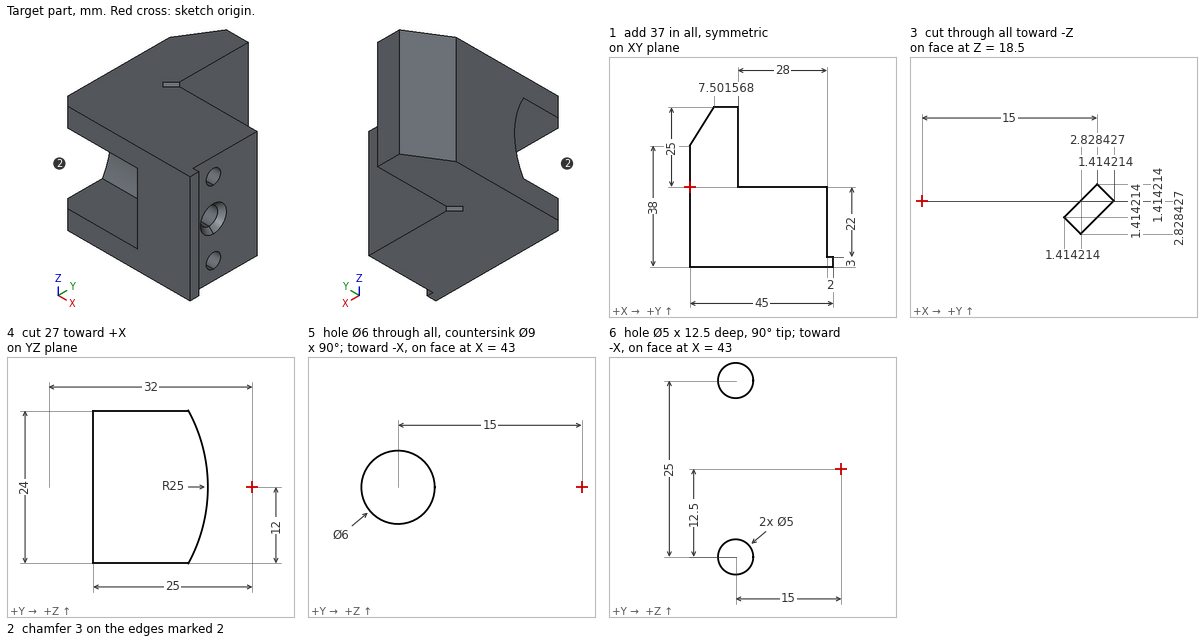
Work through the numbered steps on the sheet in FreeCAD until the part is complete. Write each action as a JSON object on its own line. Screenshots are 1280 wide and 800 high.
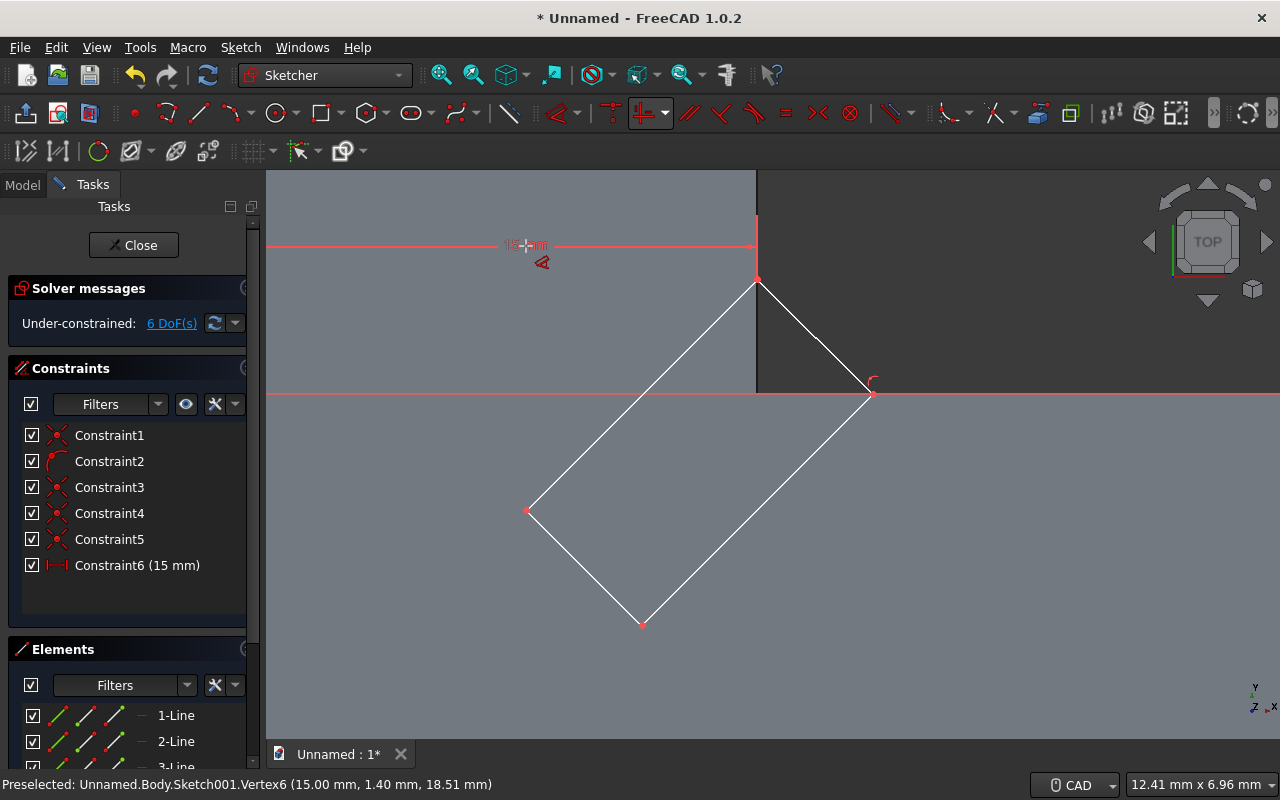
{"action": "left_click", "coordinate": [526, 511]}
{"action": "left_click", "coordinate": [560, 453]}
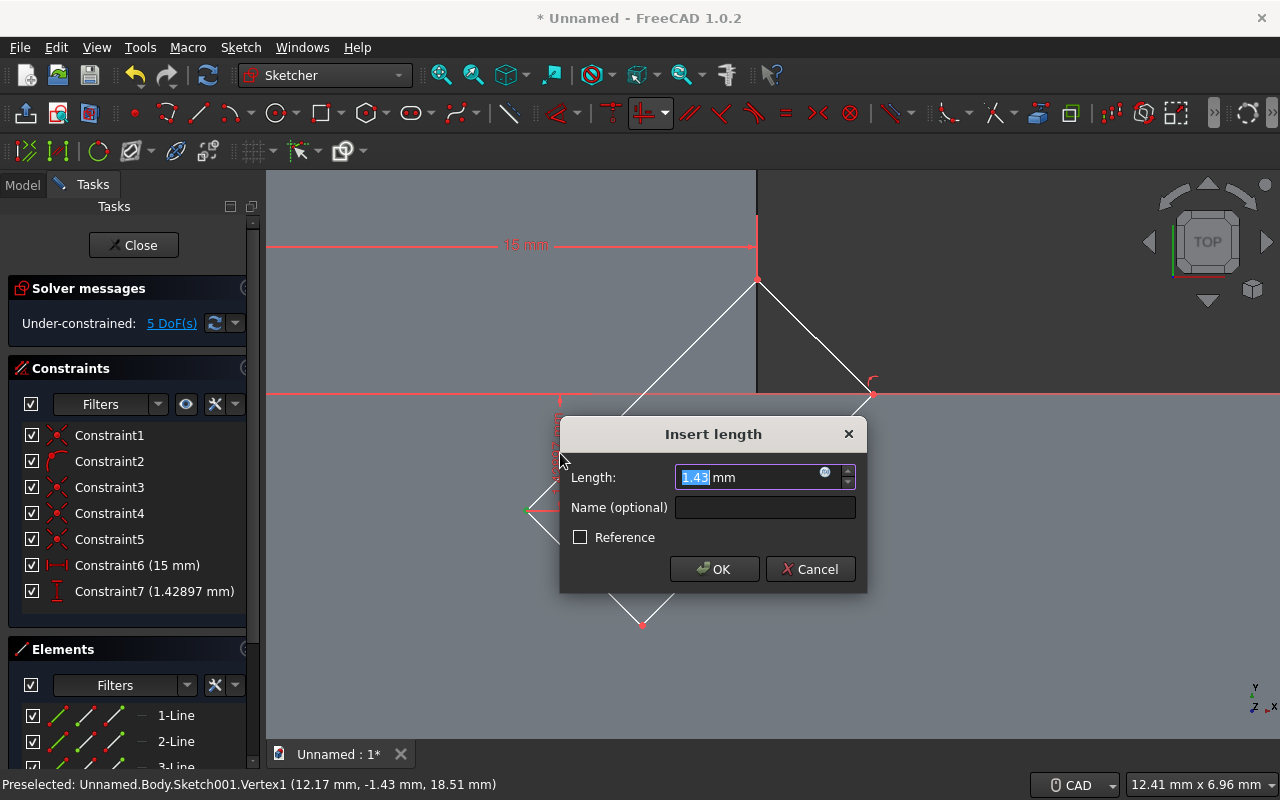
{"action": "type", "text": "1.414214"}
{"action": "key", "text": "Return"}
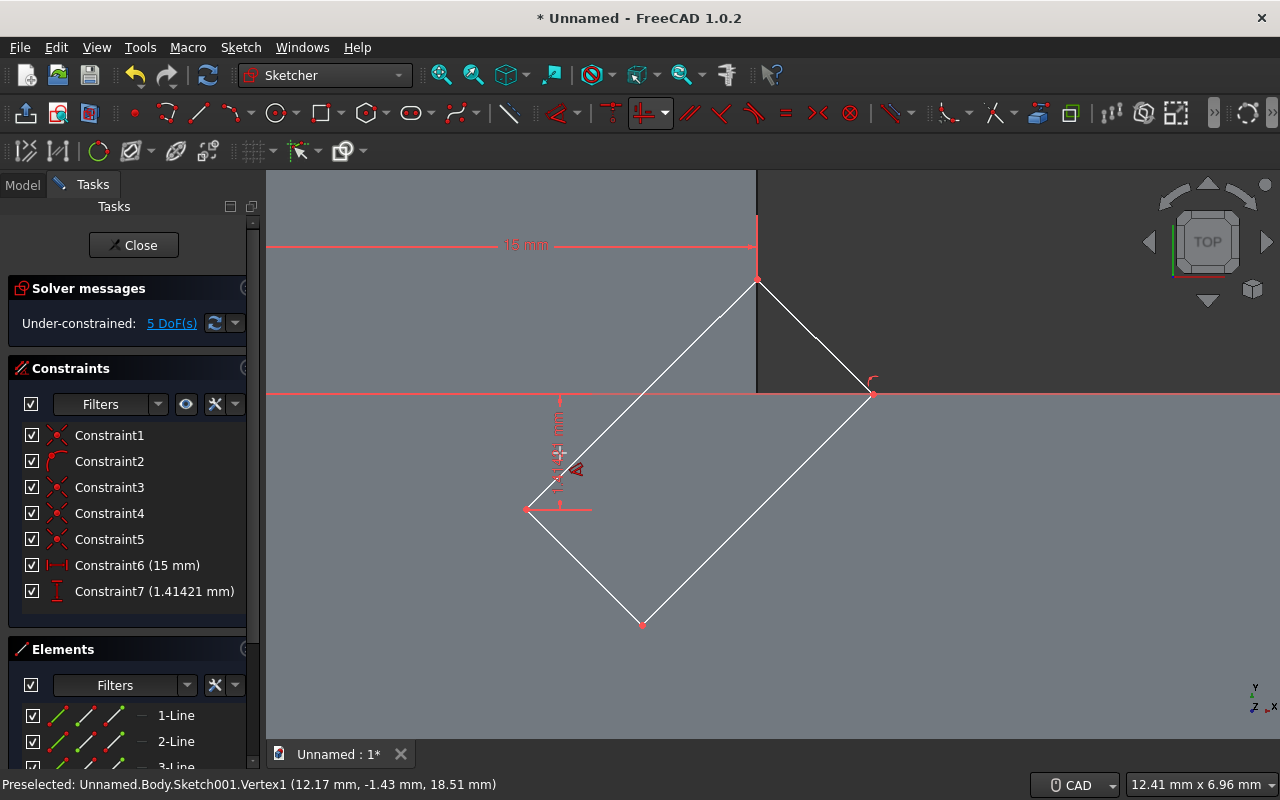
{"action": "left_click", "coordinate": [642, 626]}
{"action": "left_click", "coordinate": [676, 510]}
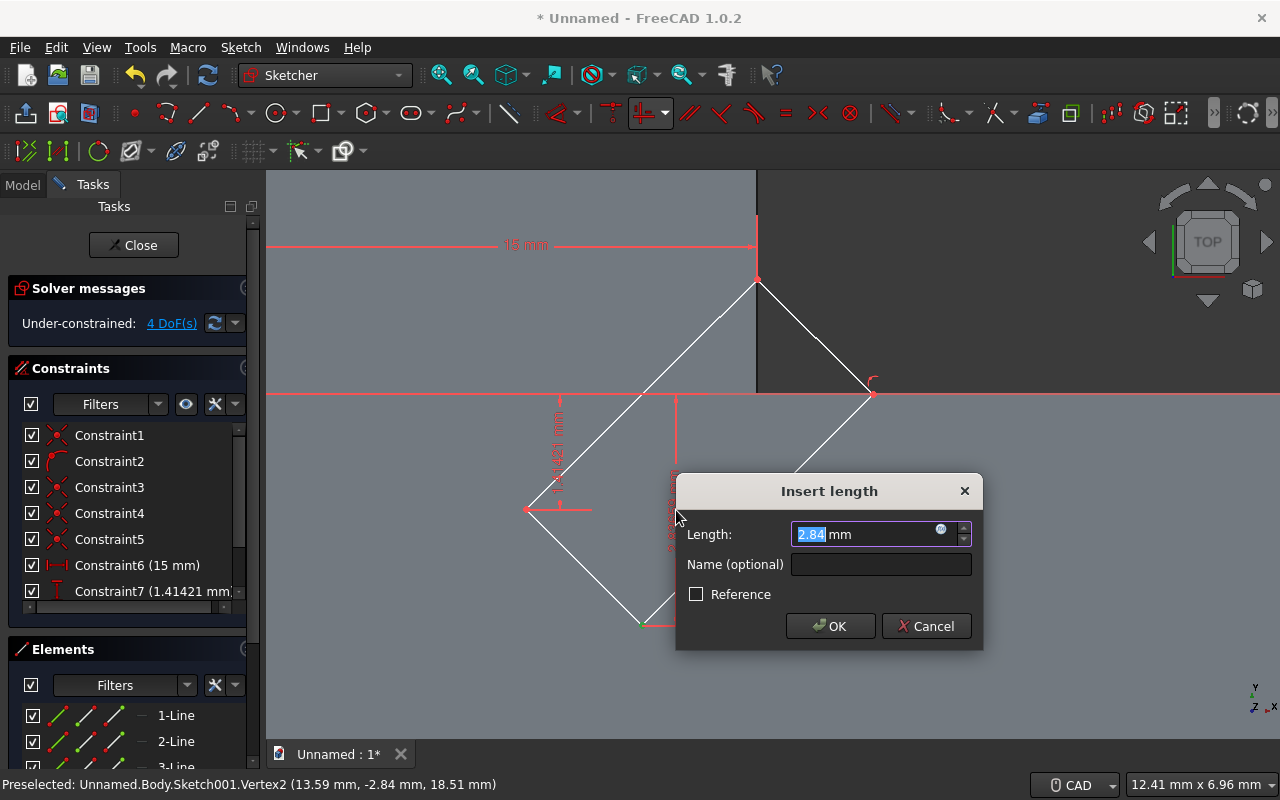
{"action": "type", "text": "2.828427"}
{"action": "key", "text": "Return"}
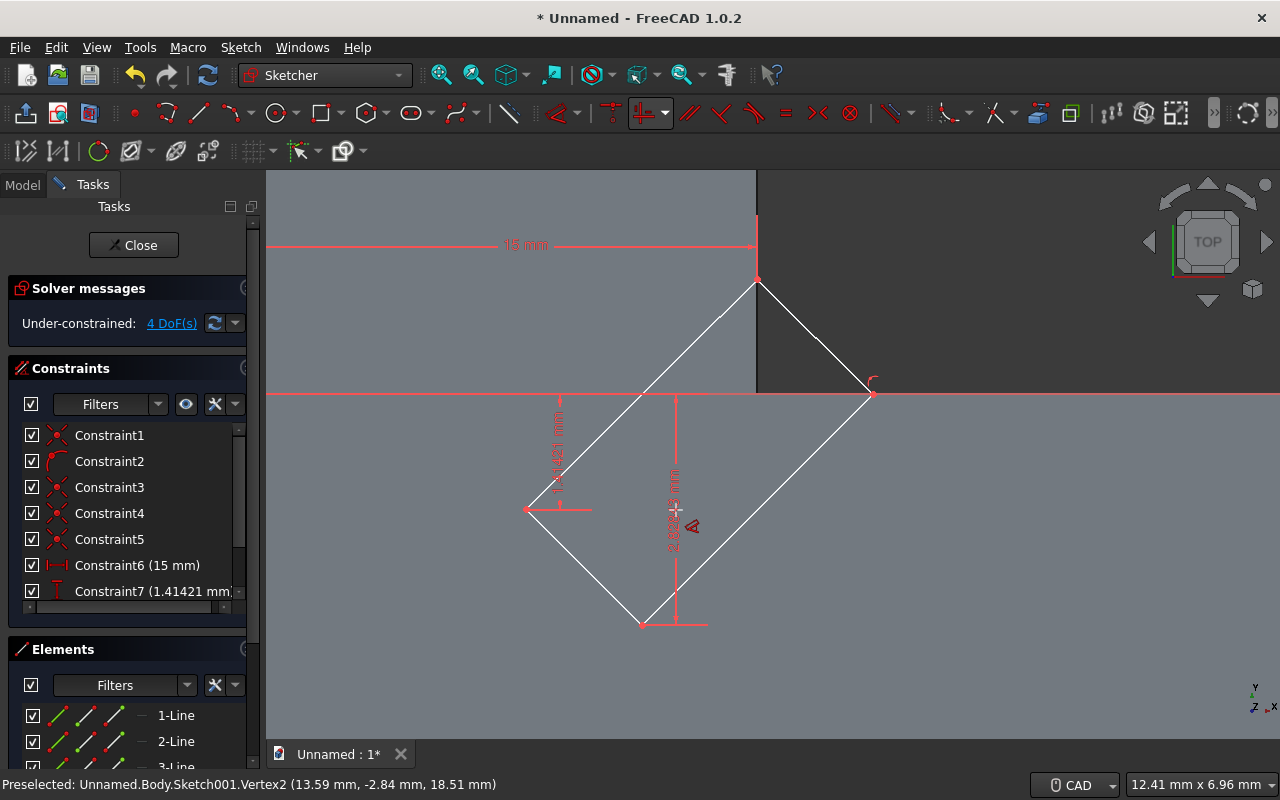
{"action": "left_click", "coordinate": [757, 280]}
{"action": "left_click", "coordinate": [791, 337]}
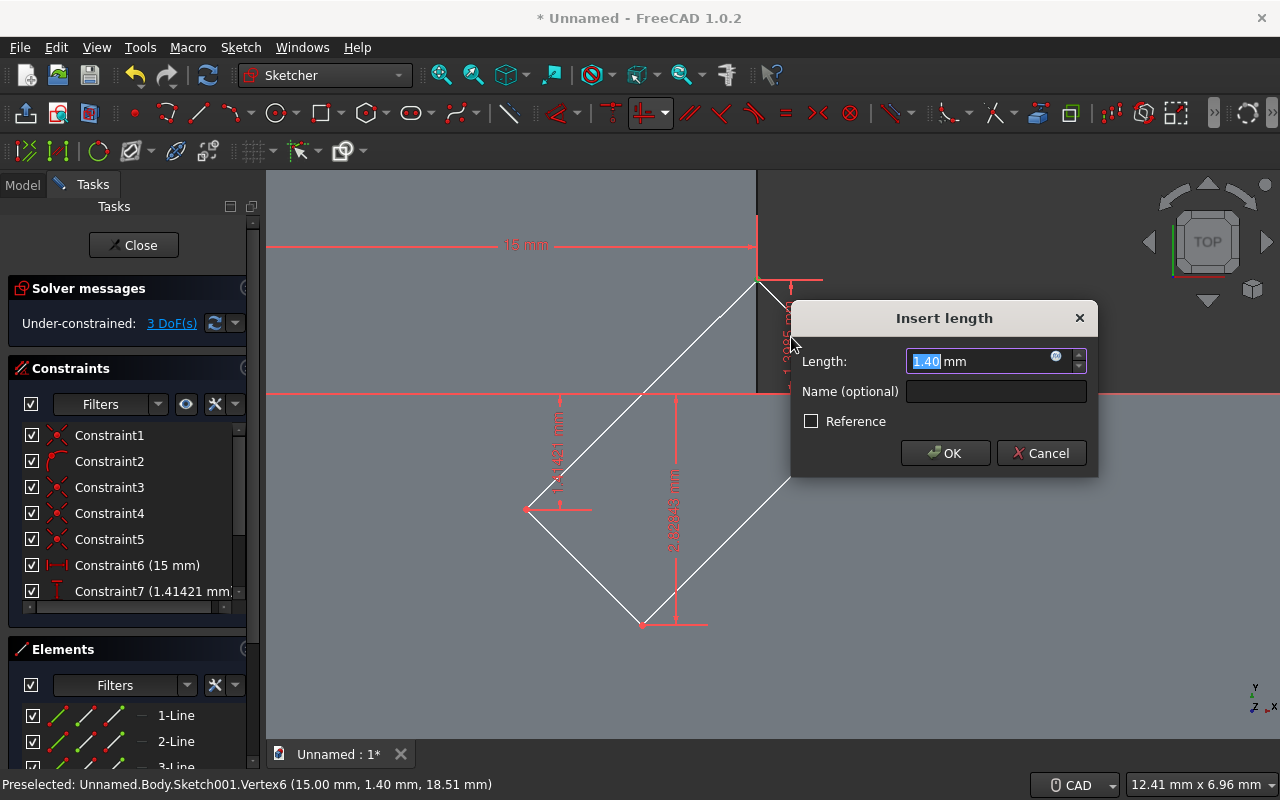
{"action": "type", "text": "1.414214"}
{"action": "key", "text": "Return"}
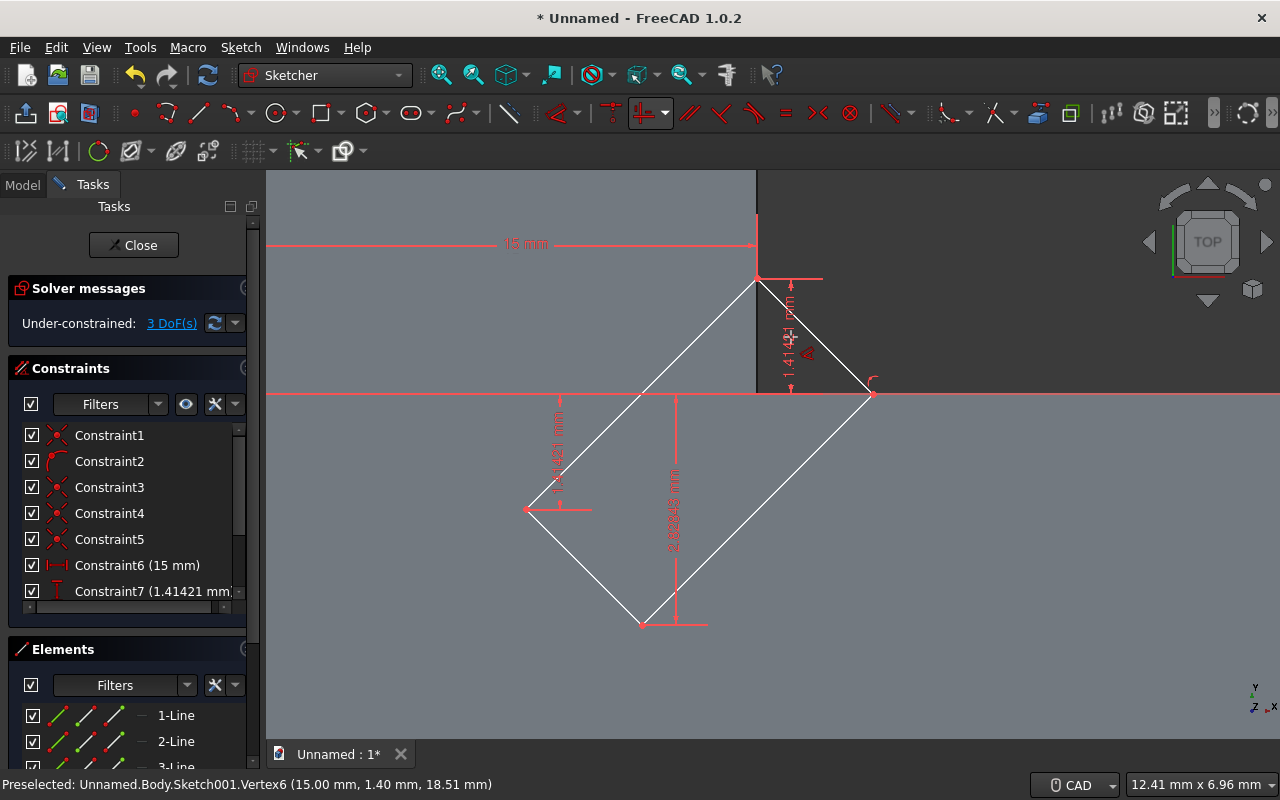
{"action": "left_click", "coordinate": [561, 544]}
{"action": "left_click", "coordinate": [584, 659]}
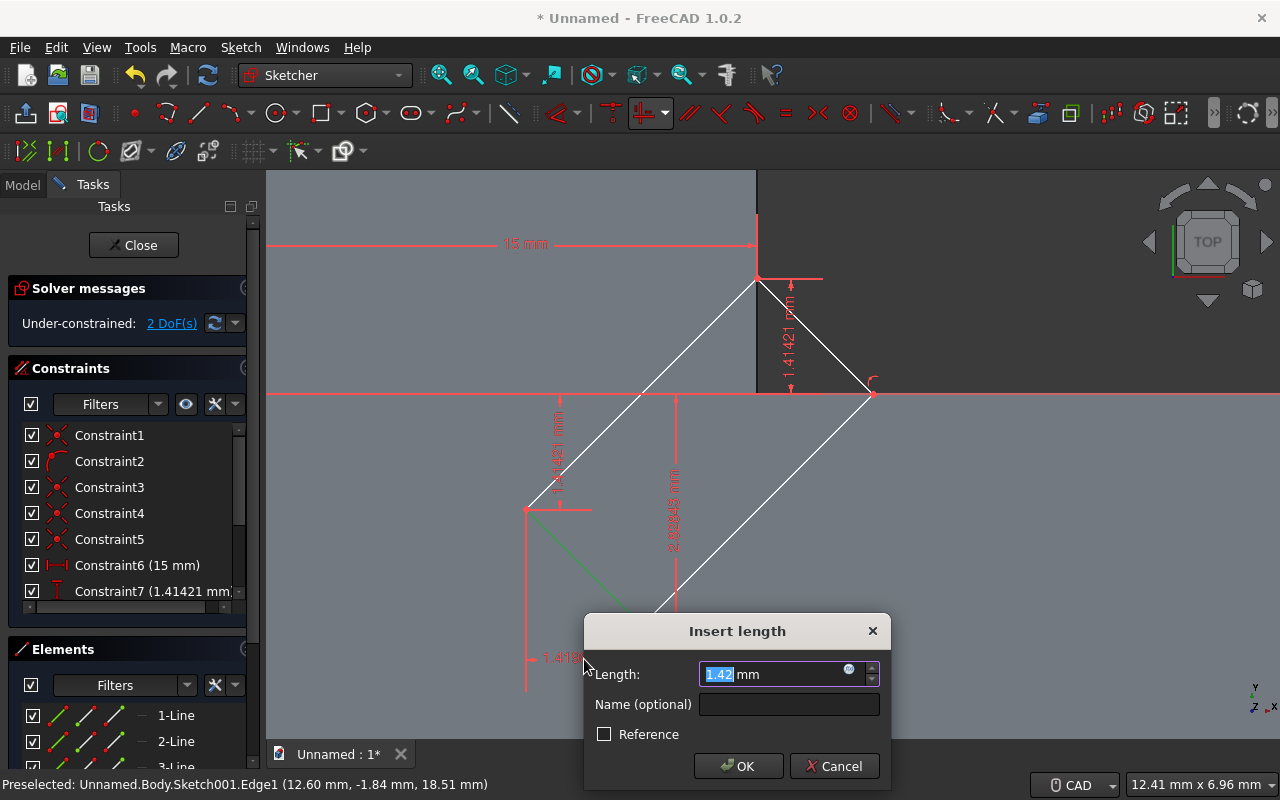
{"action": "type", "text": "1.414214"}
{"action": "key", "text": "Return"}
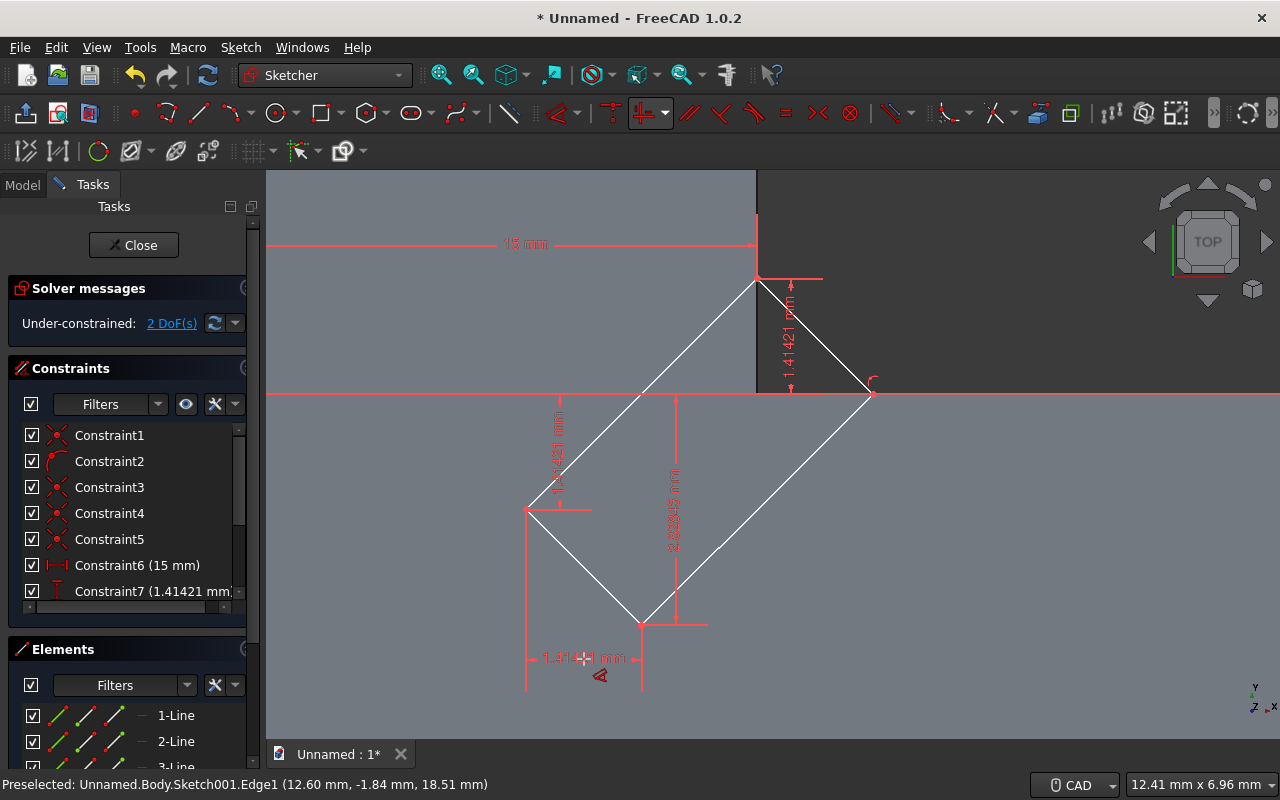
{"action": "left_click", "coordinate": [711, 556]}
{"action": "left_click", "coordinate": [757, 659]}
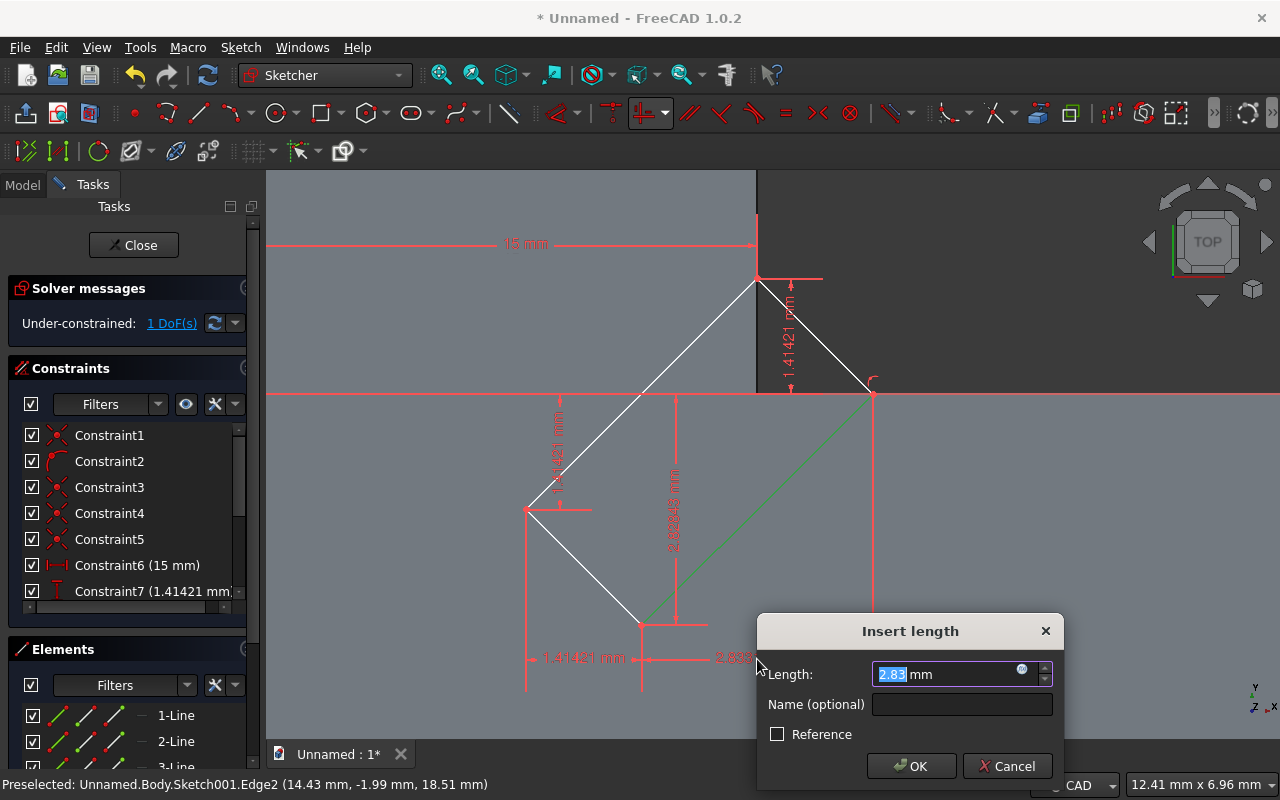
{"action": "type", "text": "2.828427"}
{"action": "key", "text": "Return"}